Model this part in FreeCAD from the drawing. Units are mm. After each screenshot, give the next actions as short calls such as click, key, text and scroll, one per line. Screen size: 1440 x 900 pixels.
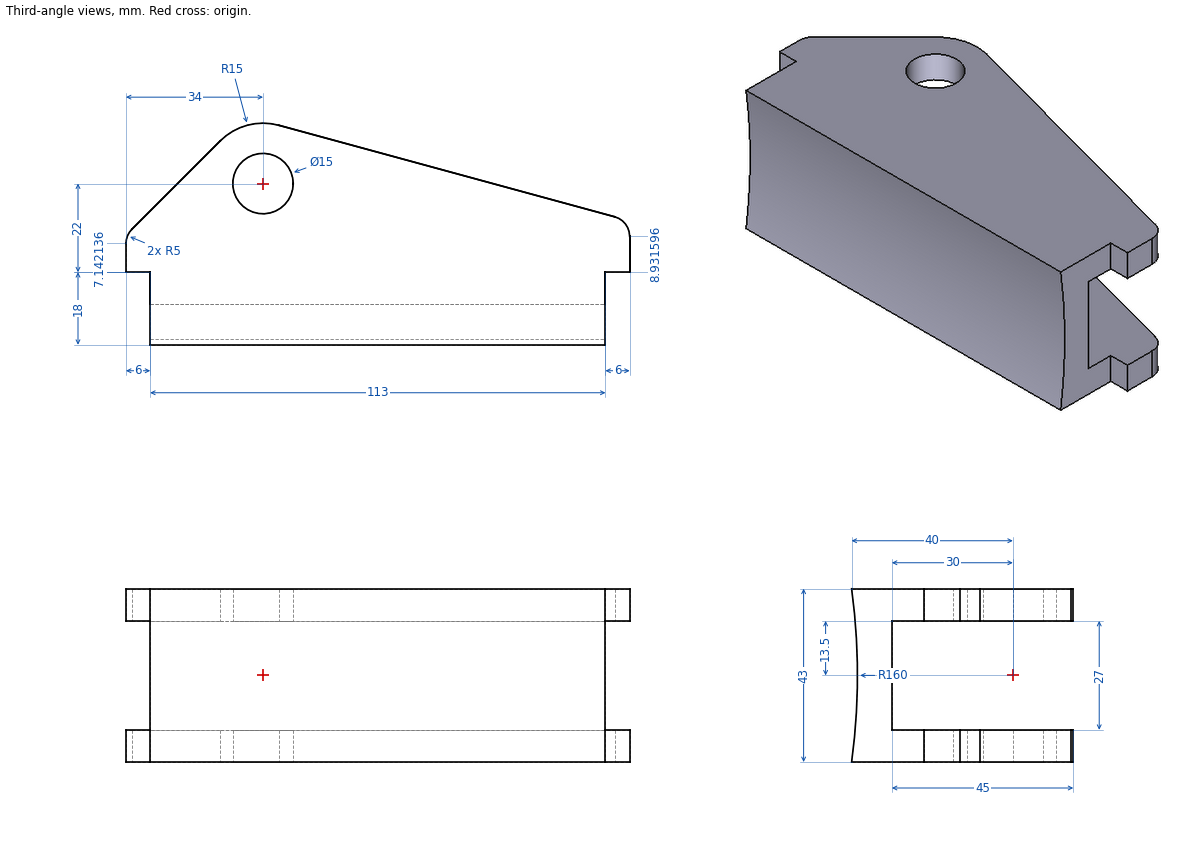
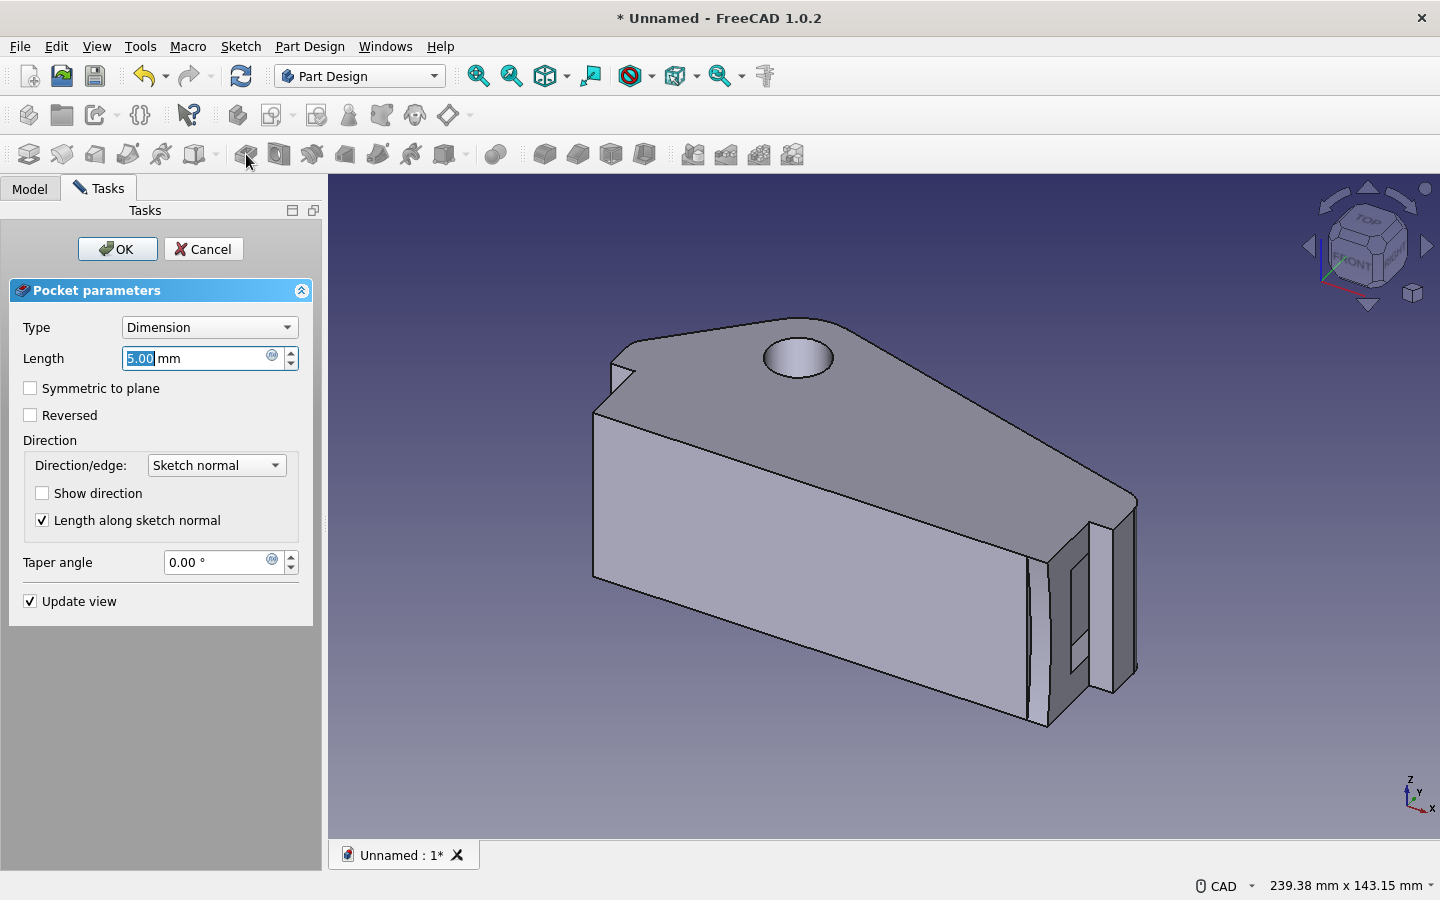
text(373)
key(Tab)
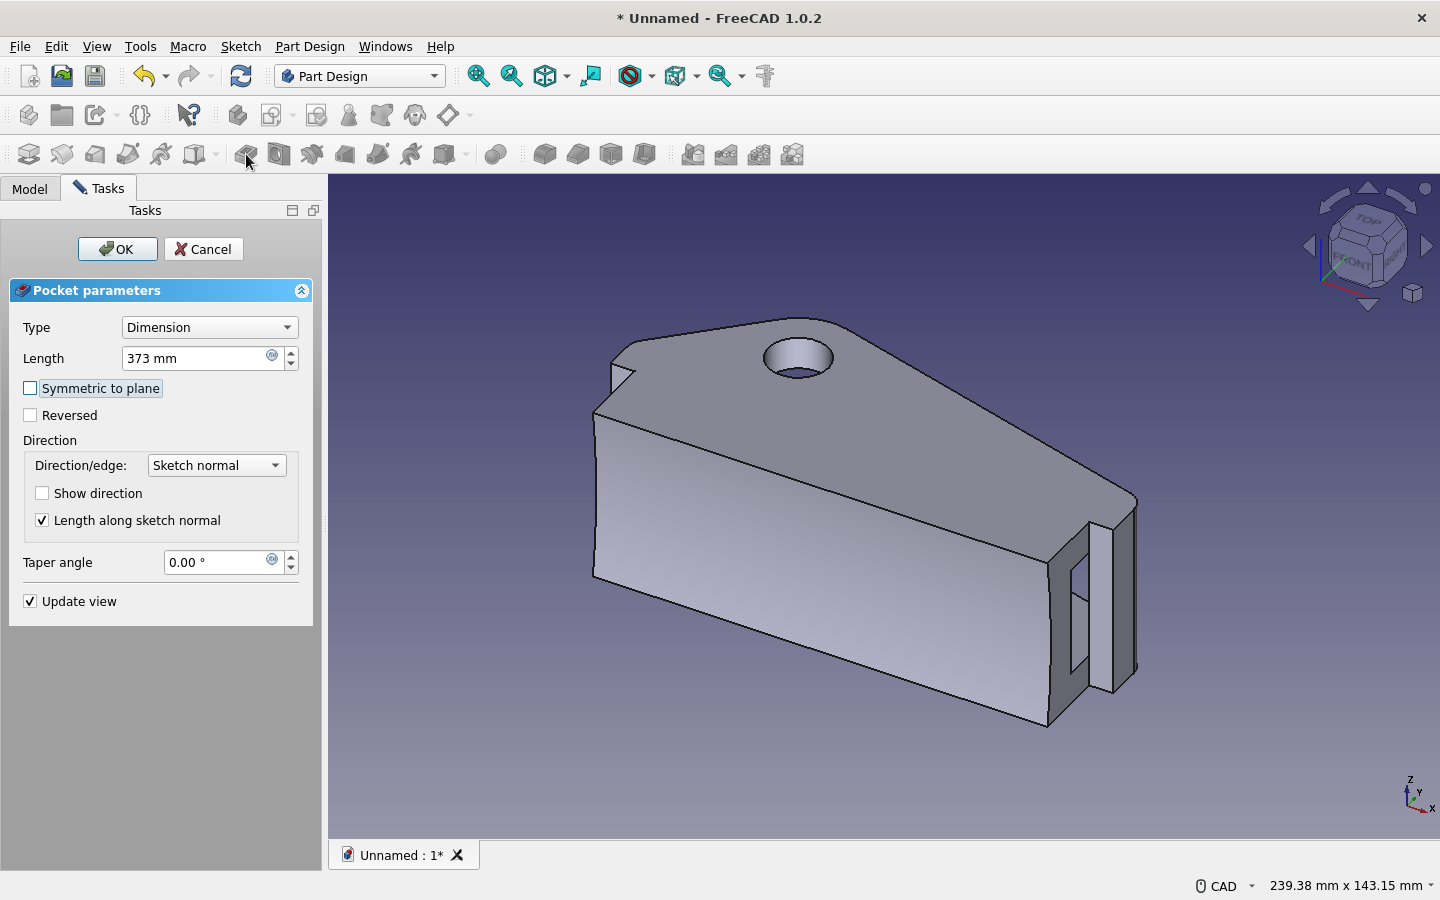
click(31, 388)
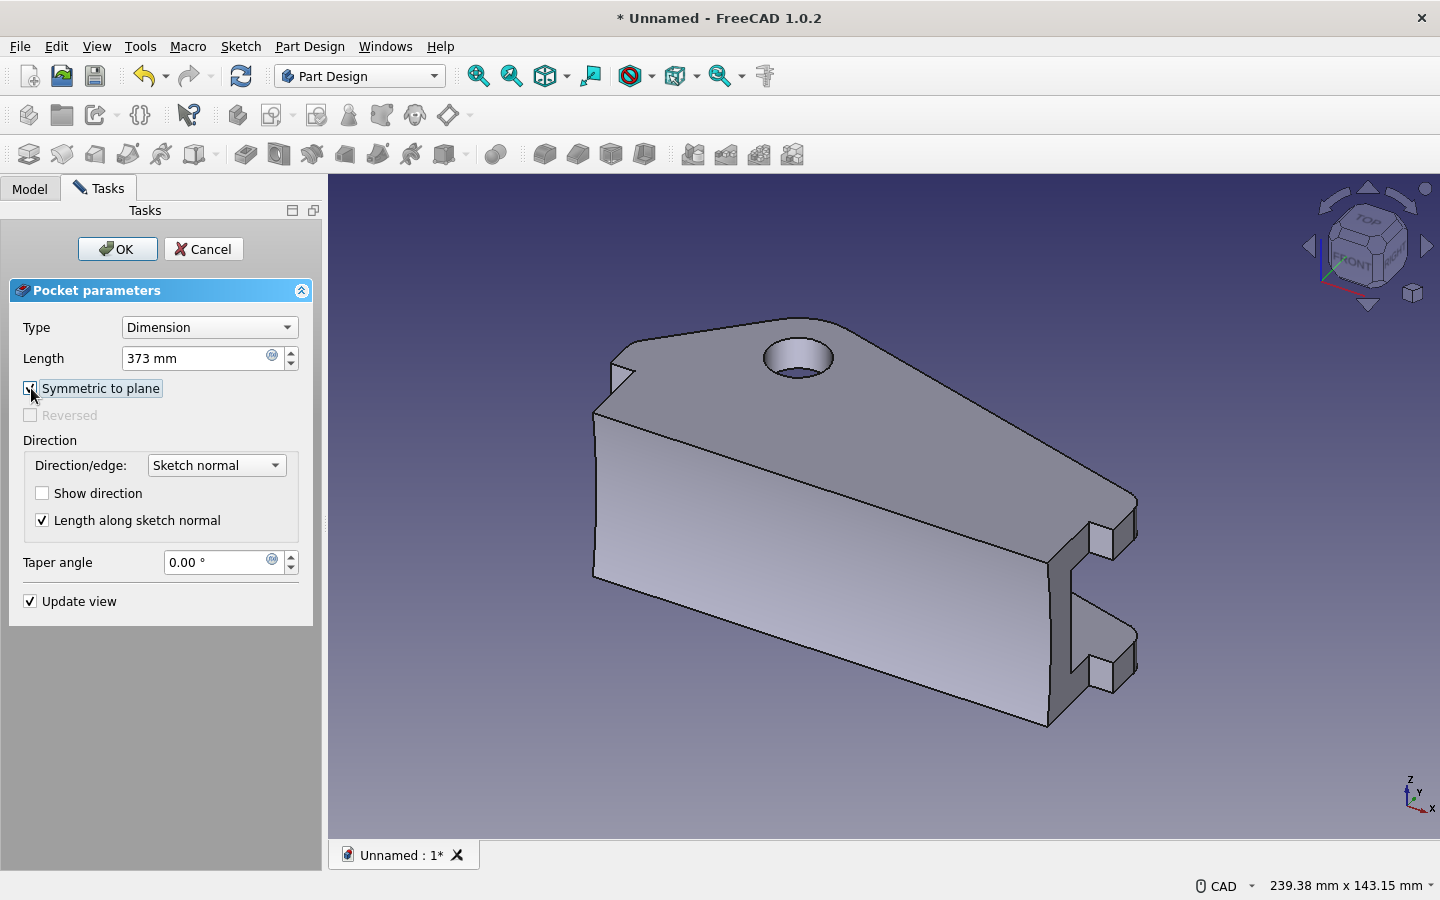
click(118, 249)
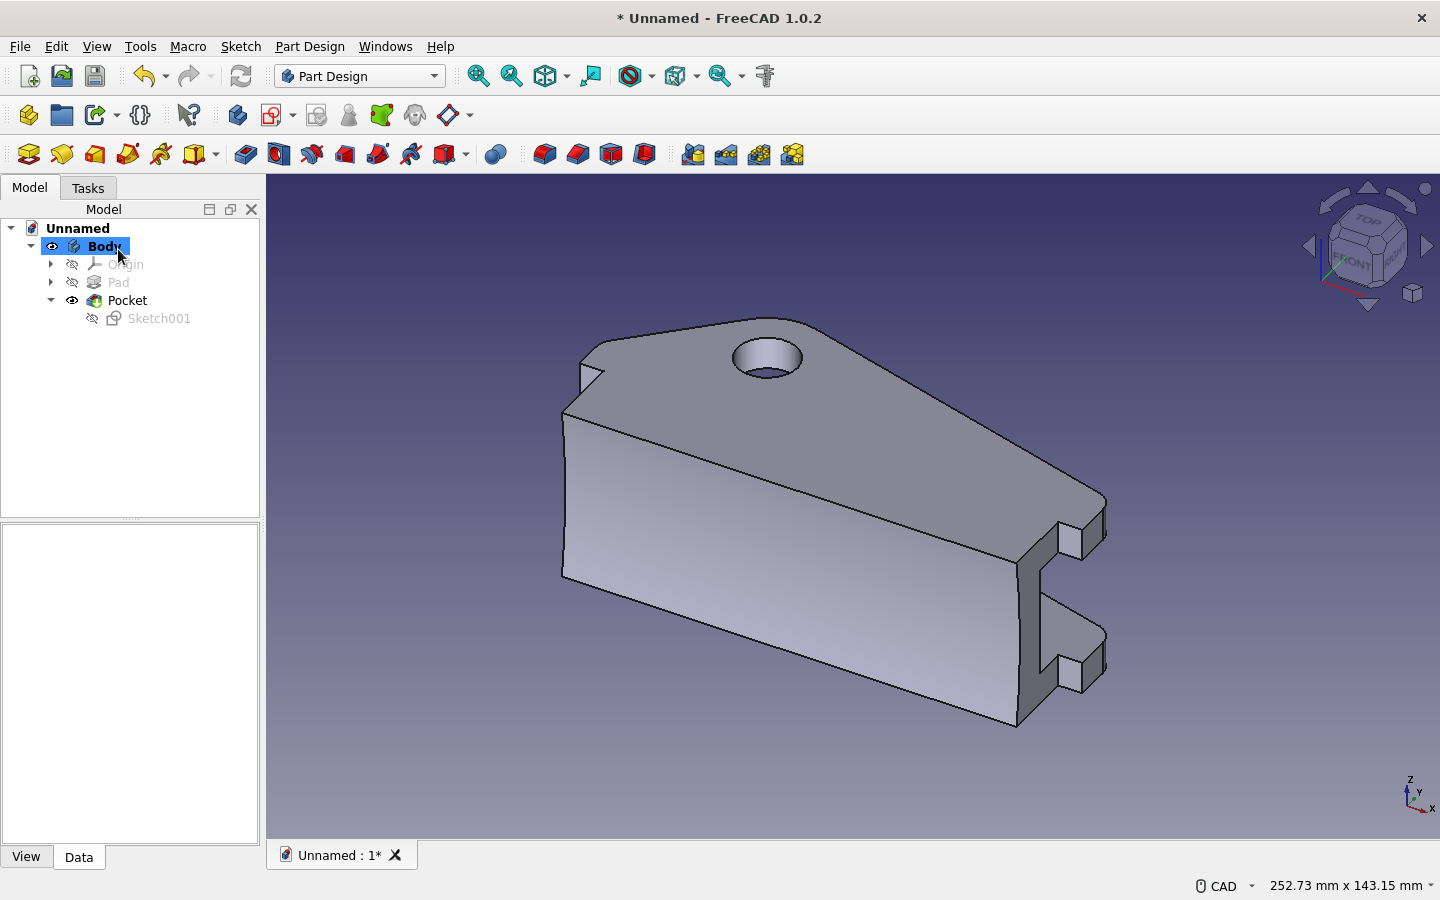
key(0)